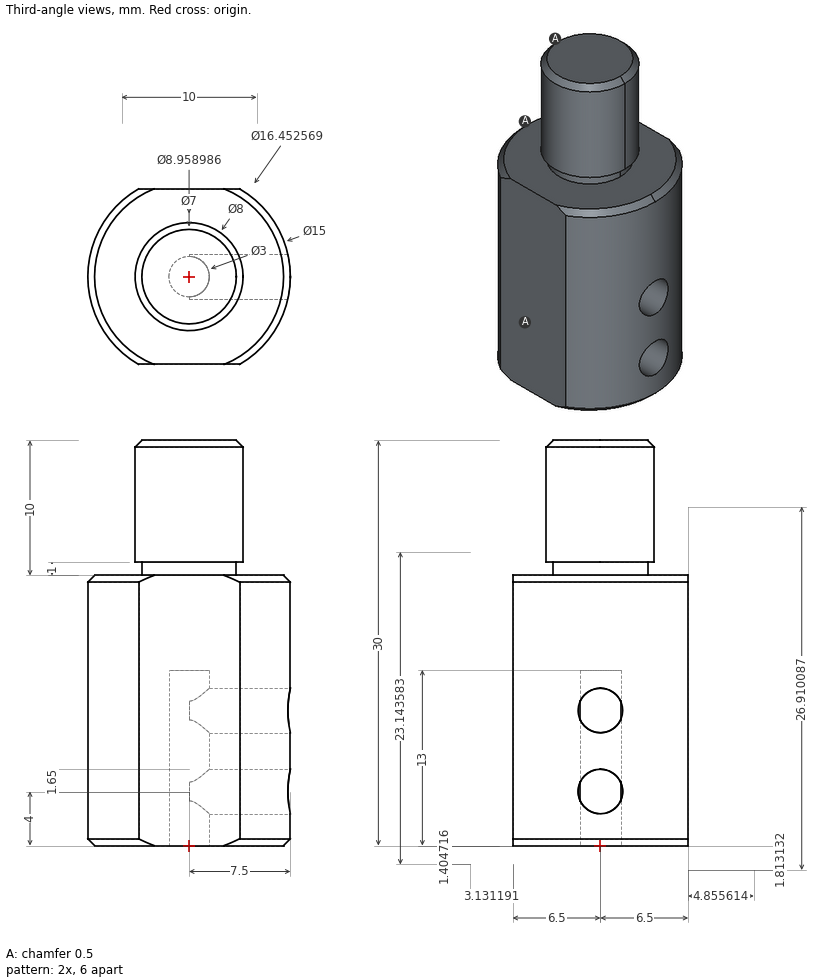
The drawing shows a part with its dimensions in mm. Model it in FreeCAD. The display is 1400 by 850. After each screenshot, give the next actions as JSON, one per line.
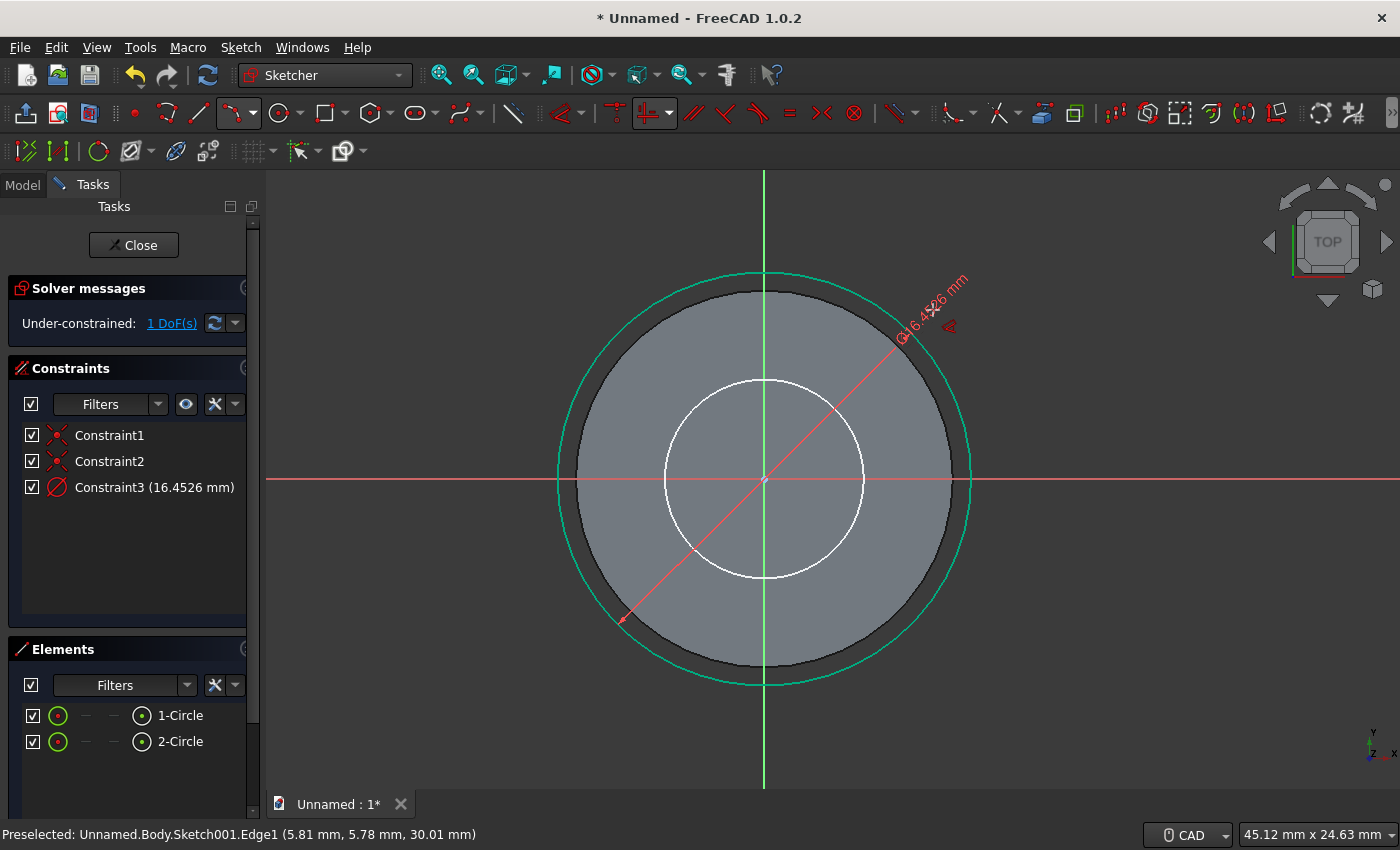
{"action": "left_click", "coordinate": [834, 408]}
{"action": "left_click", "coordinate": [856, 385]}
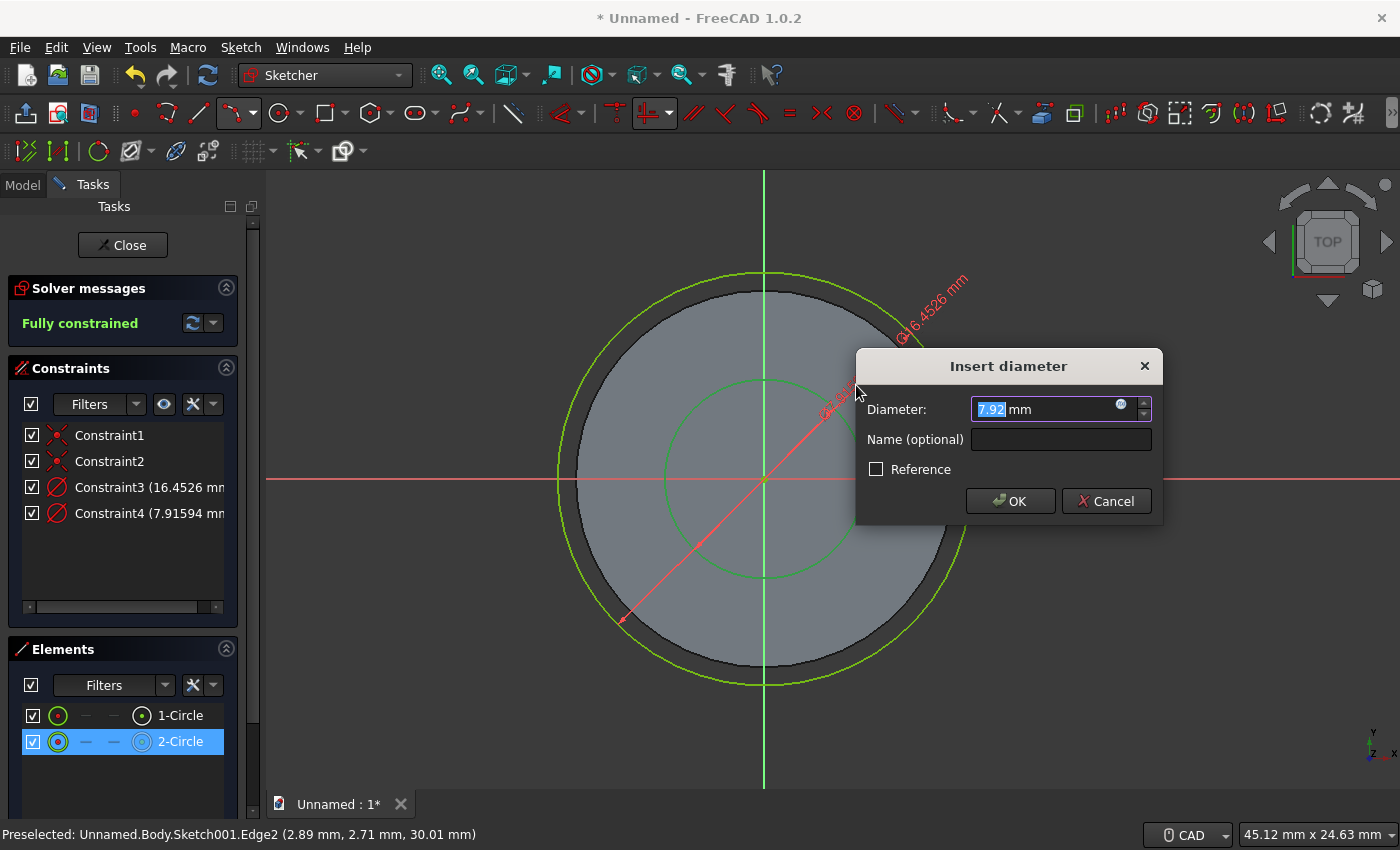
{"action": "type", "text": "8"}
{"action": "key", "text": "Return"}
{"action": "key", "text": "Escape"}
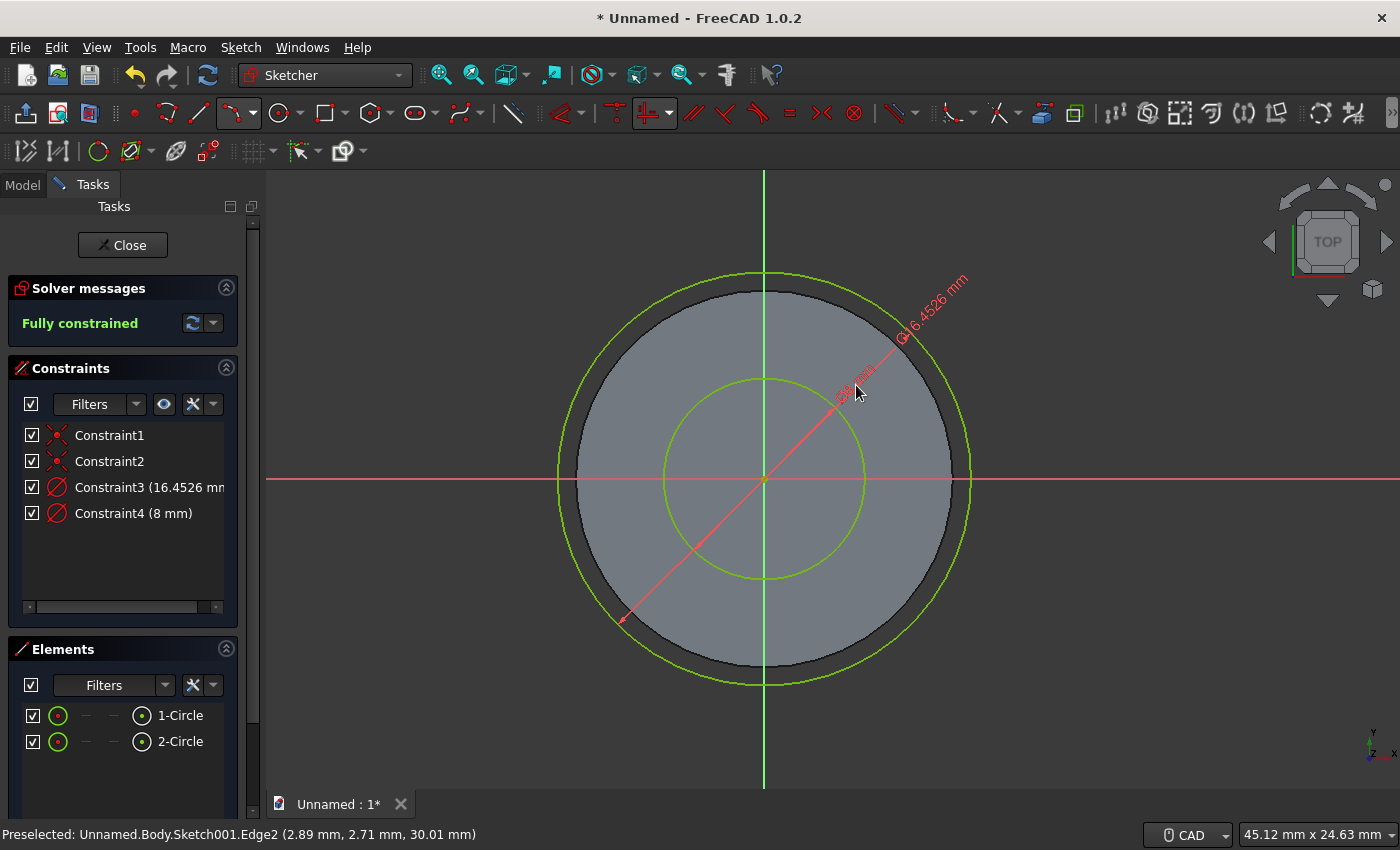
{"action": "left_click", "coordinate": [123, 245]}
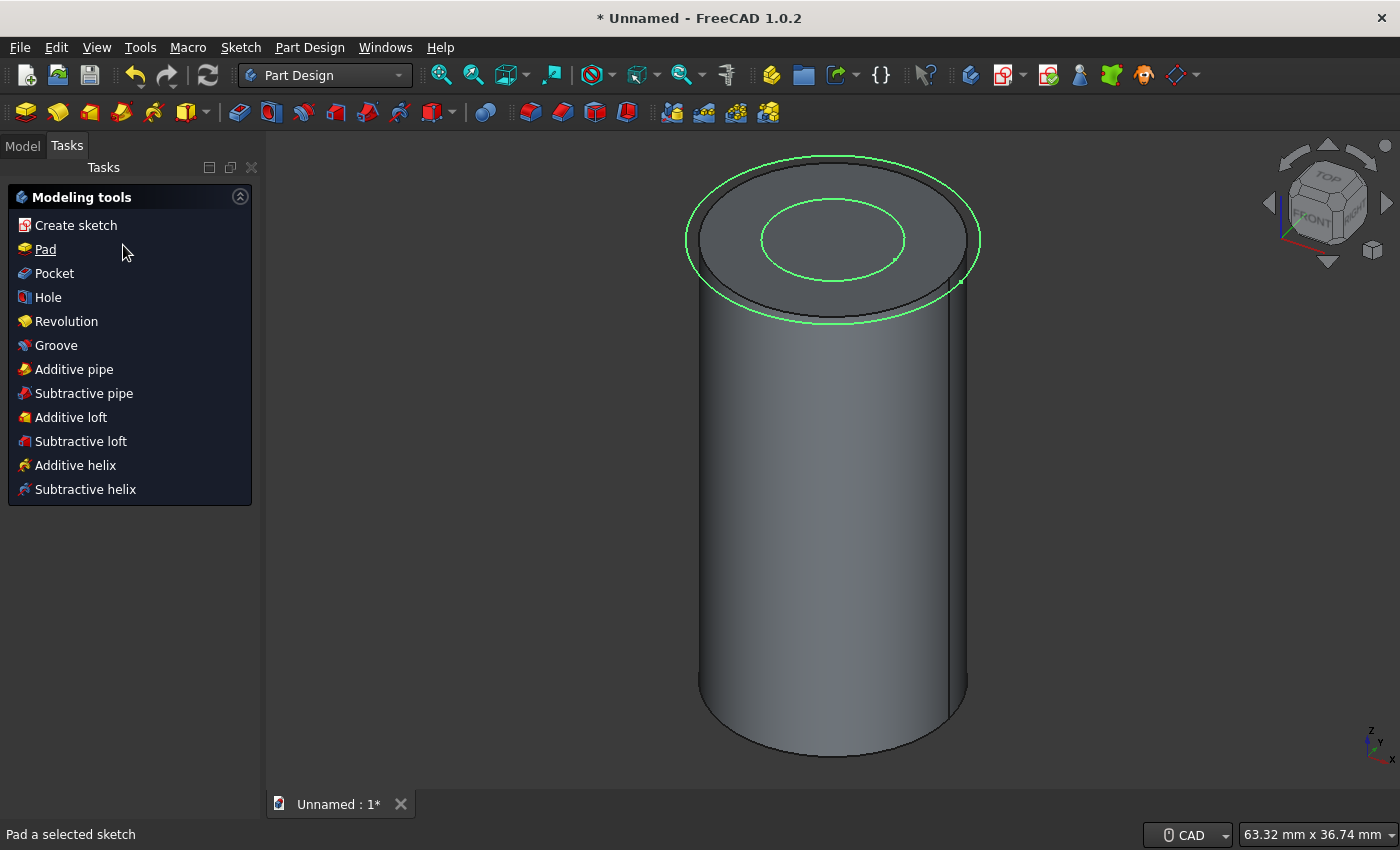
{"action": "left_click", "coordinate": [240, 112]}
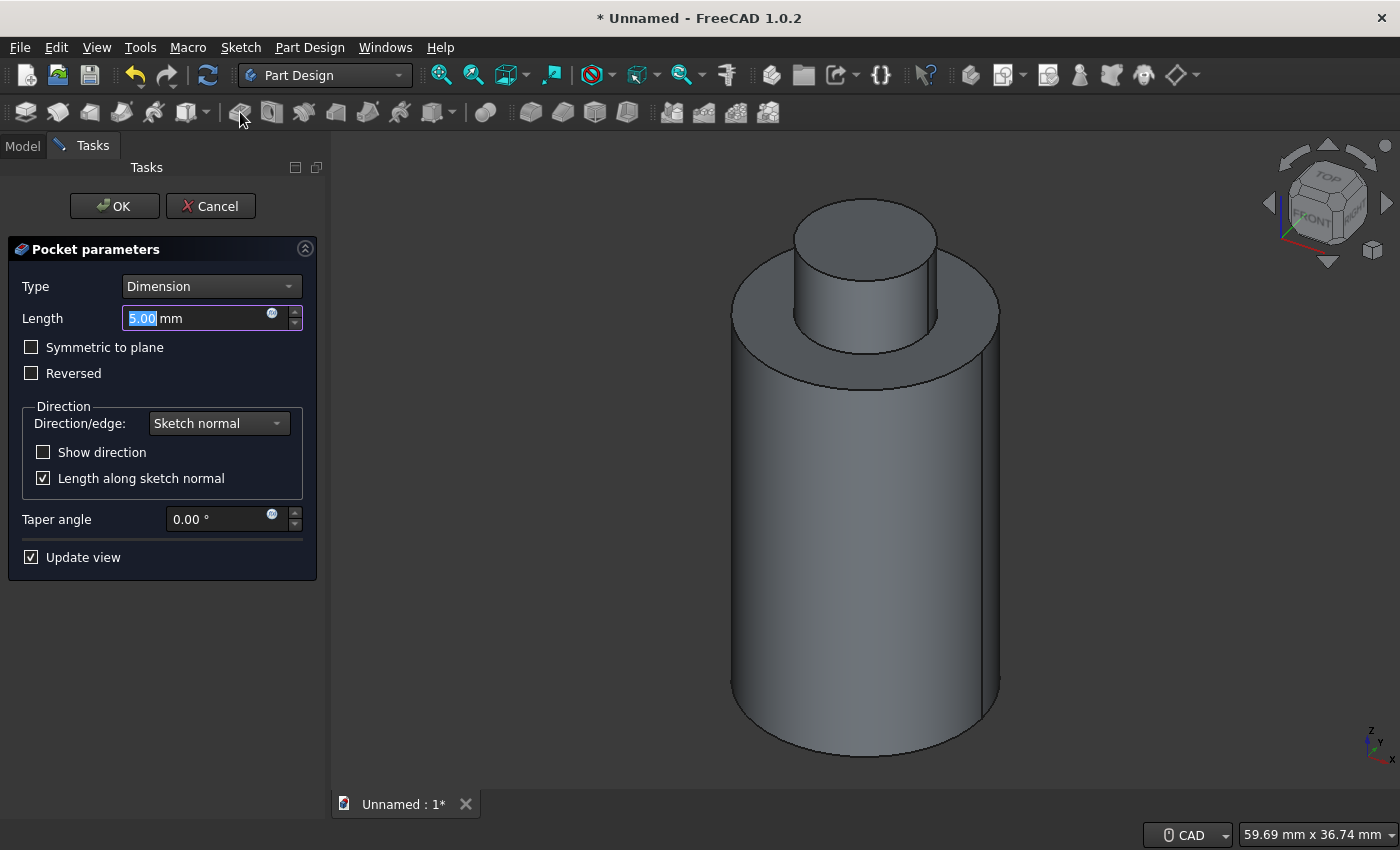
{"action": "type", "text": "10"}
{"action": "key", "text": "Tab"}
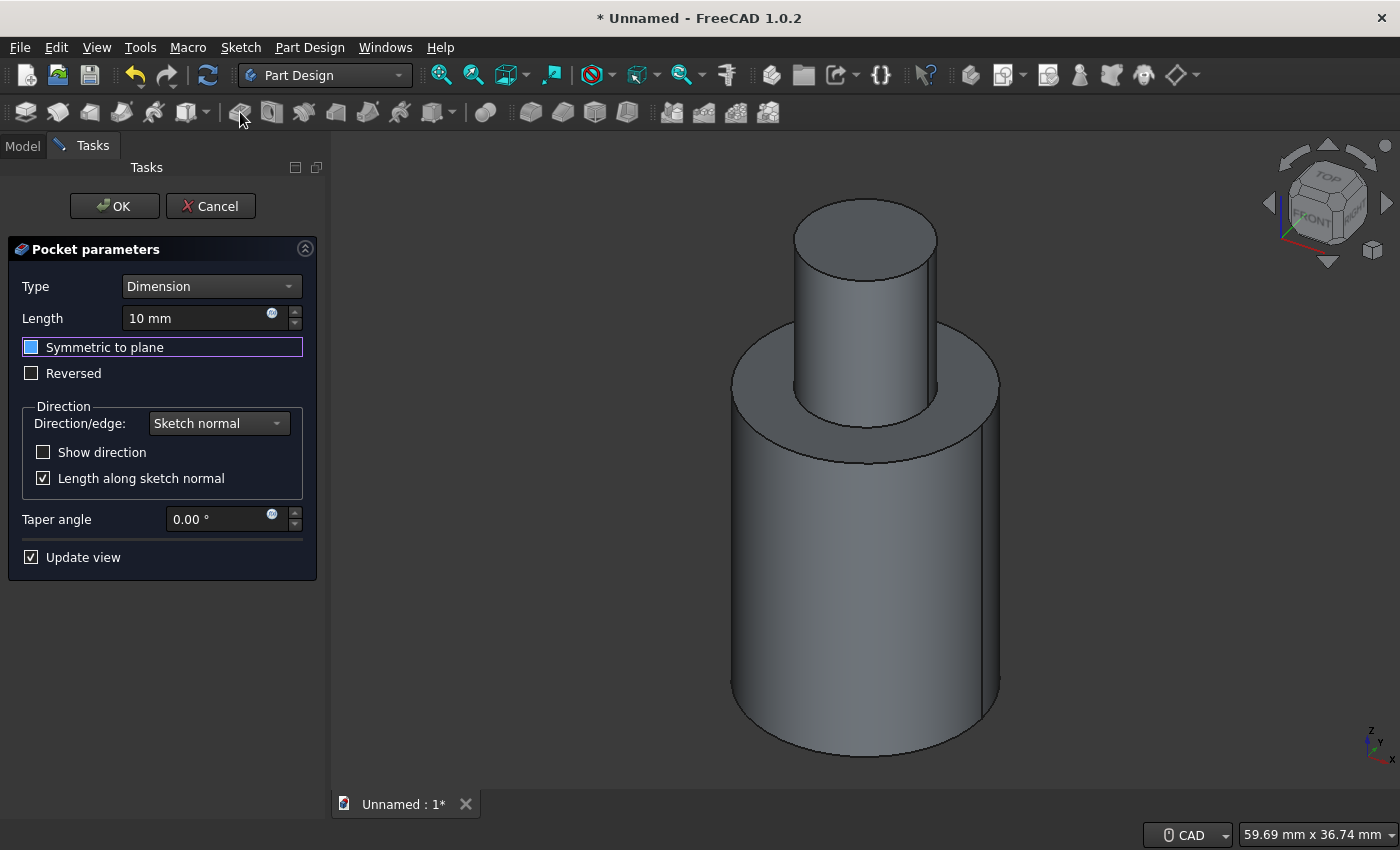
{"action": "left_click", "coordinate": [115, 206]}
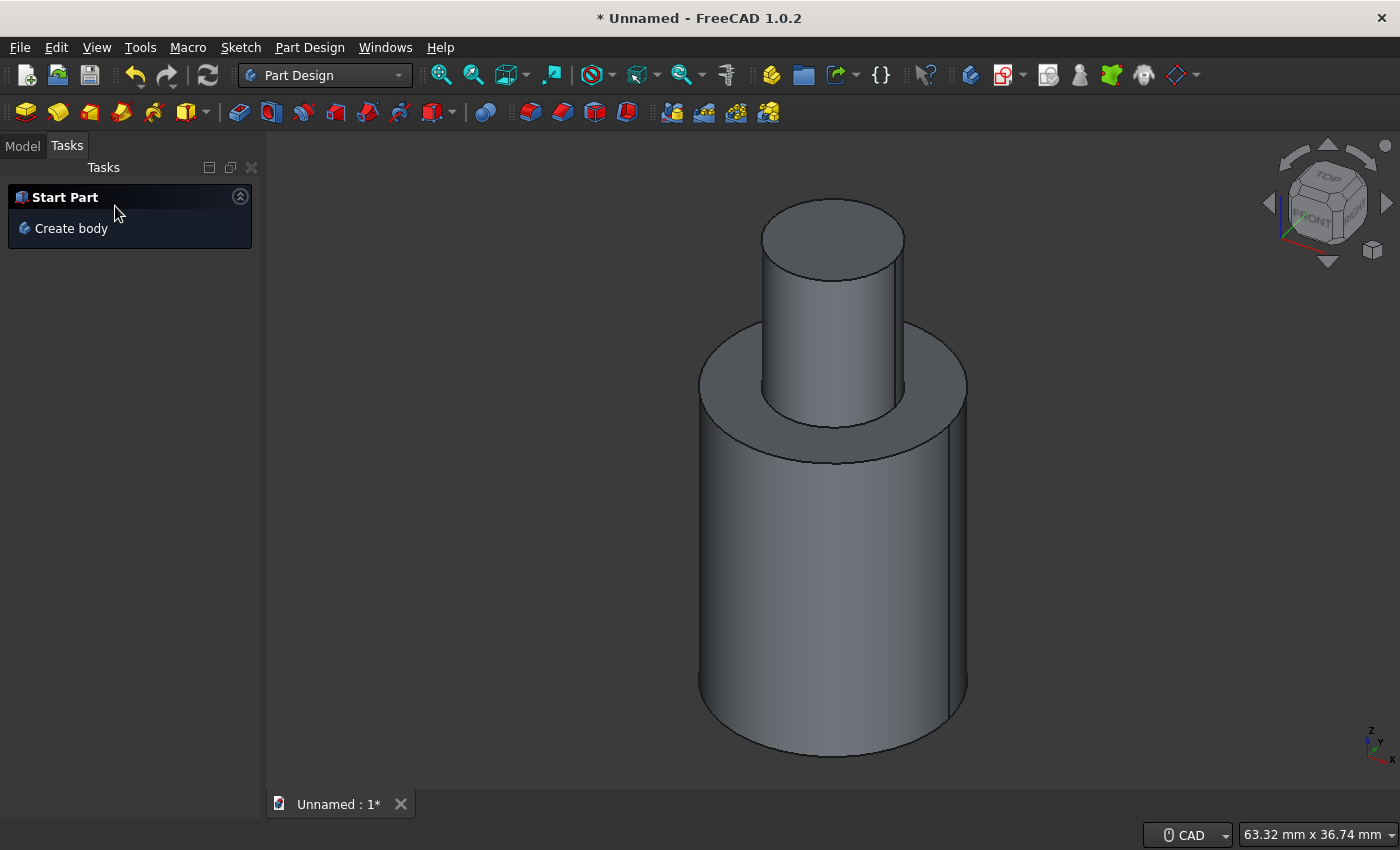
{"action": "key", "text": "5"}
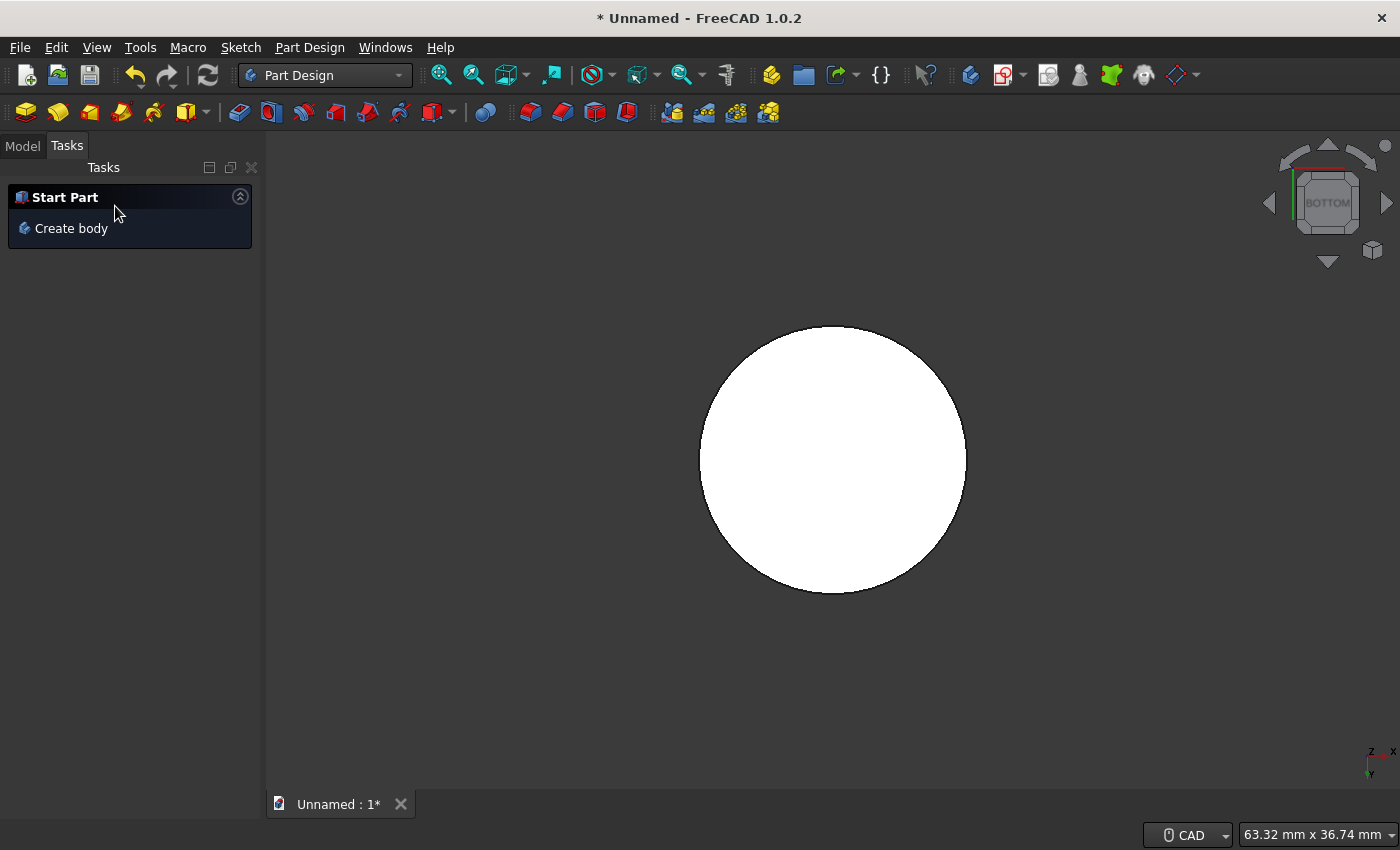
{"action": "left_click", "coordinate": [442, 76]}